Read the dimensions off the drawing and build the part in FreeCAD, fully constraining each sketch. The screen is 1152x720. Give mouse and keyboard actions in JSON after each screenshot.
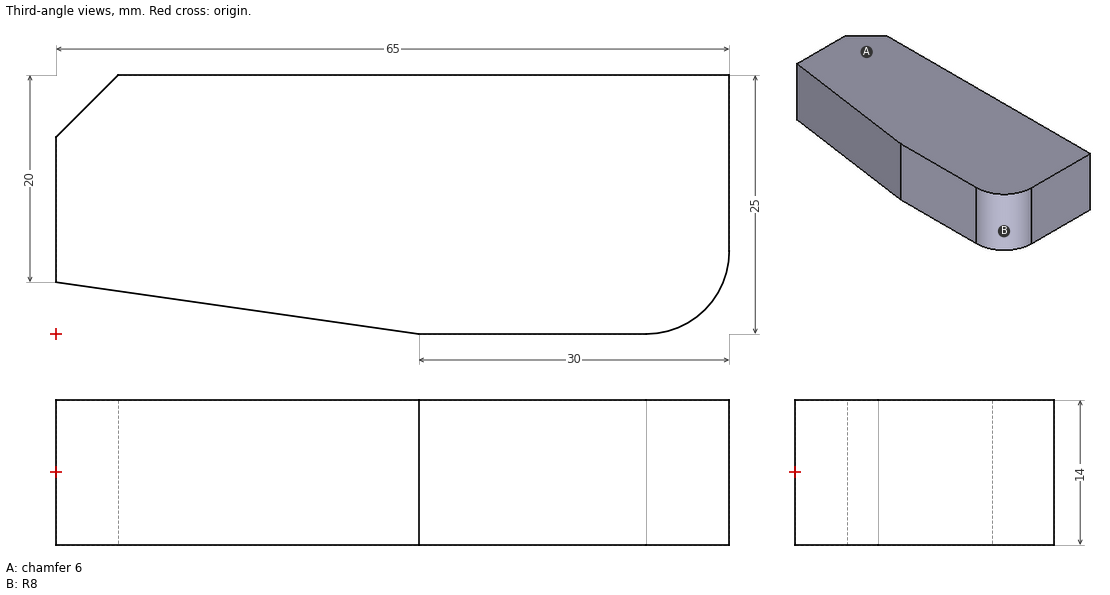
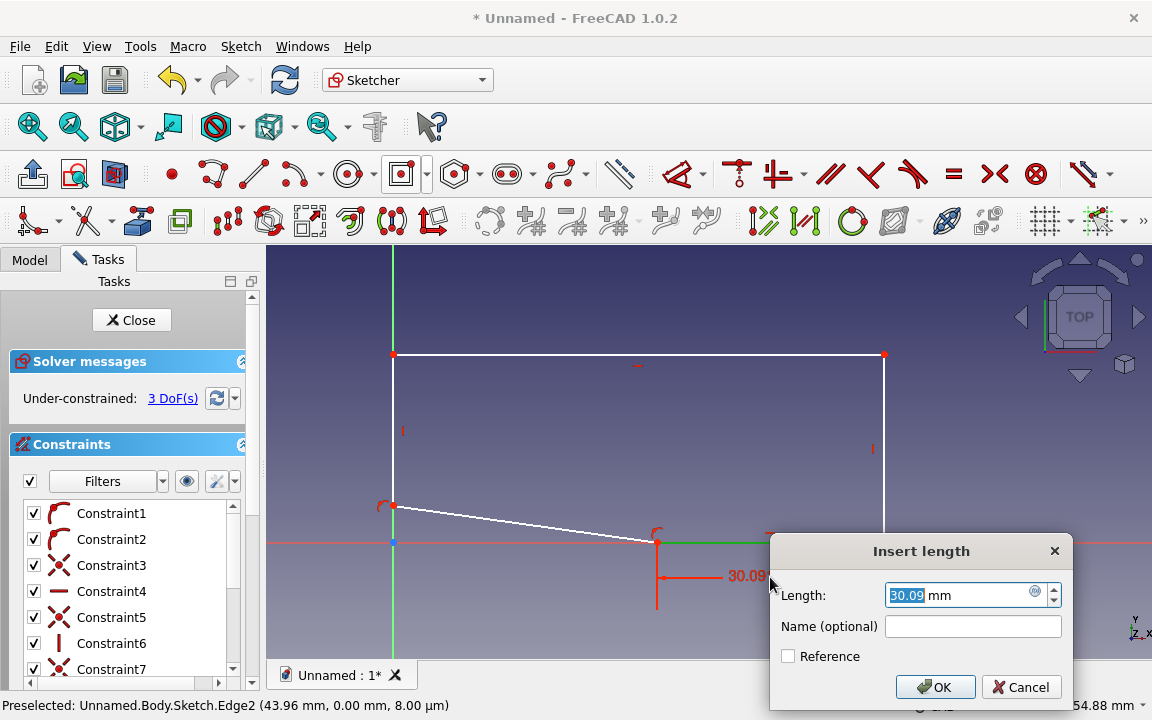
{"action": "type", "text": "30"}
{"action": "key", "text": "Return"}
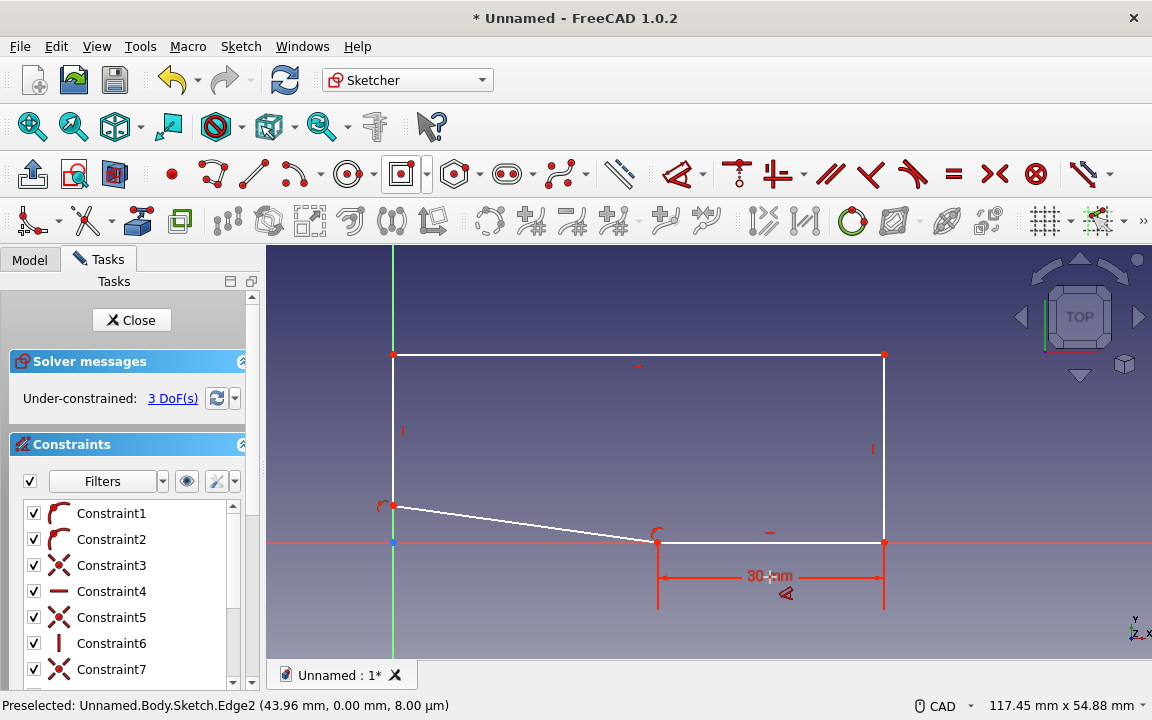
{"action": "left_click", "coordinate": [884, 486]}
{"action": "left_click", "coordinate": [918, 449]}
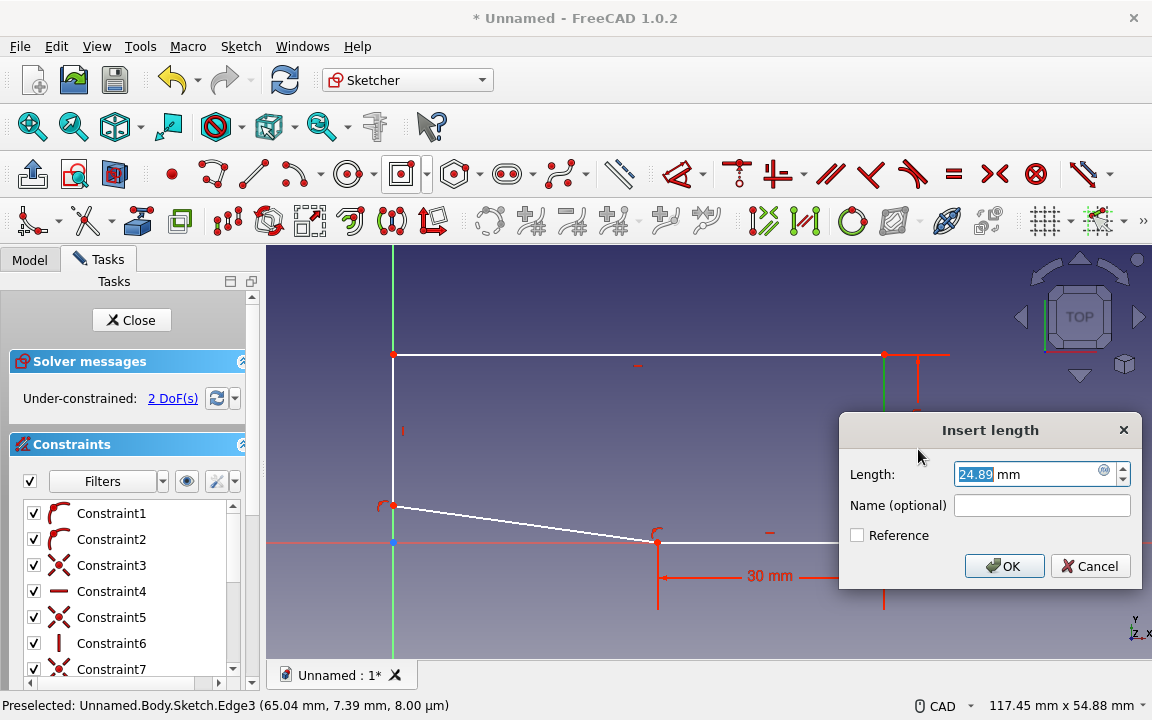
{"action": "type", "text": "25"}
{"action": "key", "text": "Return"}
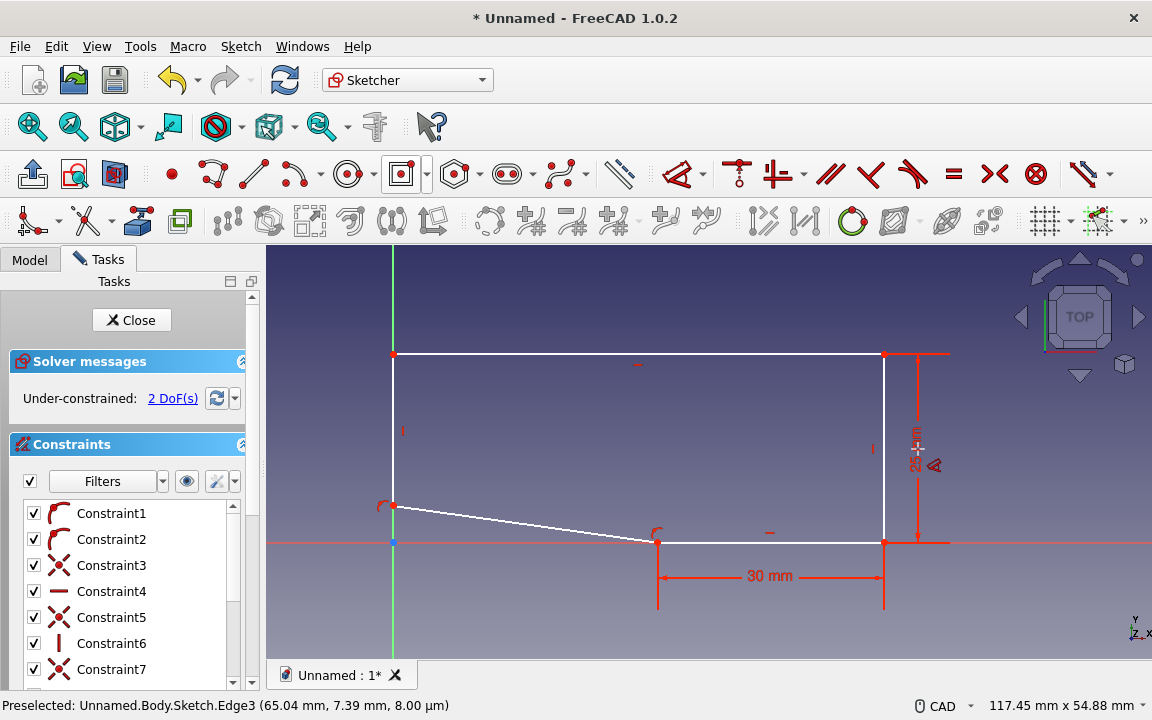
{"action": "left_click", "coordinate": [737, 354]}
{"action": "left_click", "coordinate": [639, 320]}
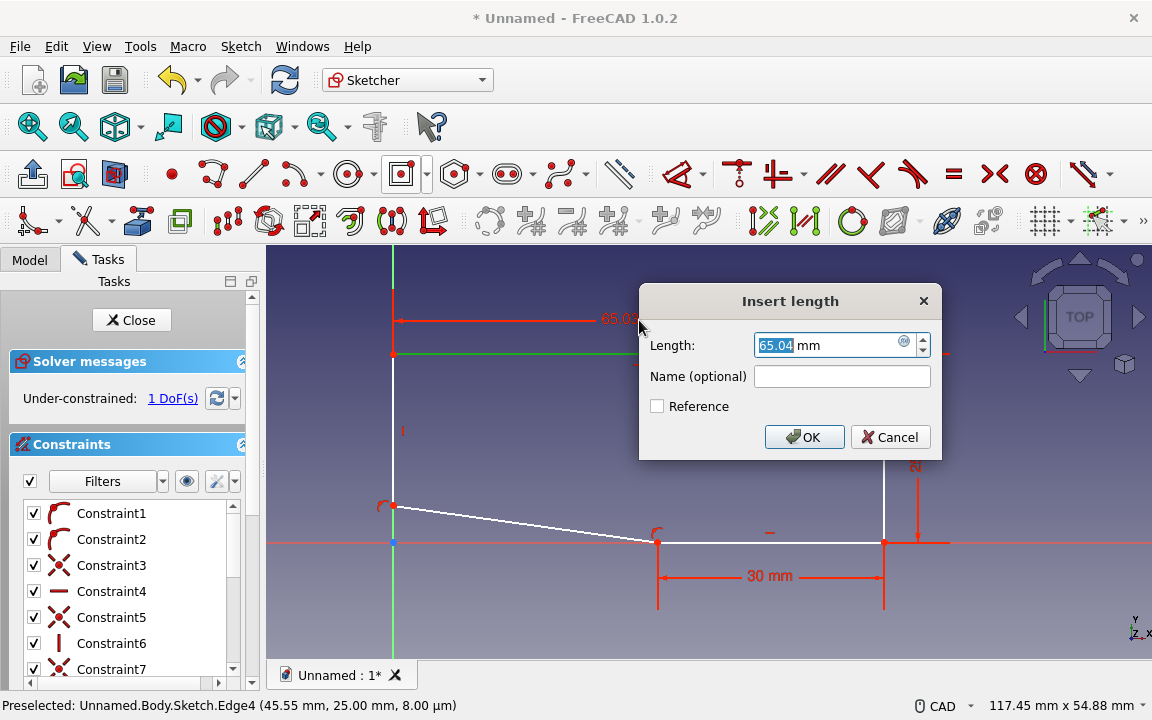
{"action": "type", "text": "65"}
{"action": "key", "text": "Return"}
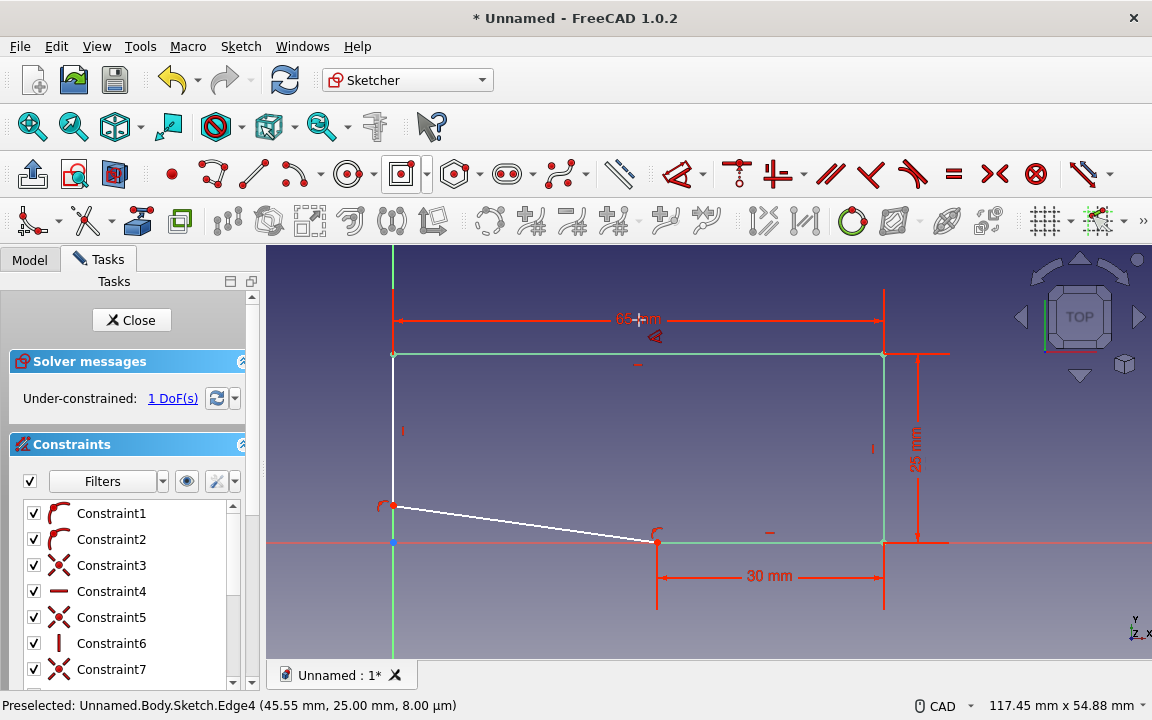
{"action": "left_click", "coordinate": [393, 400]}
{"action": "left_click", "coordinate": [359, 430]}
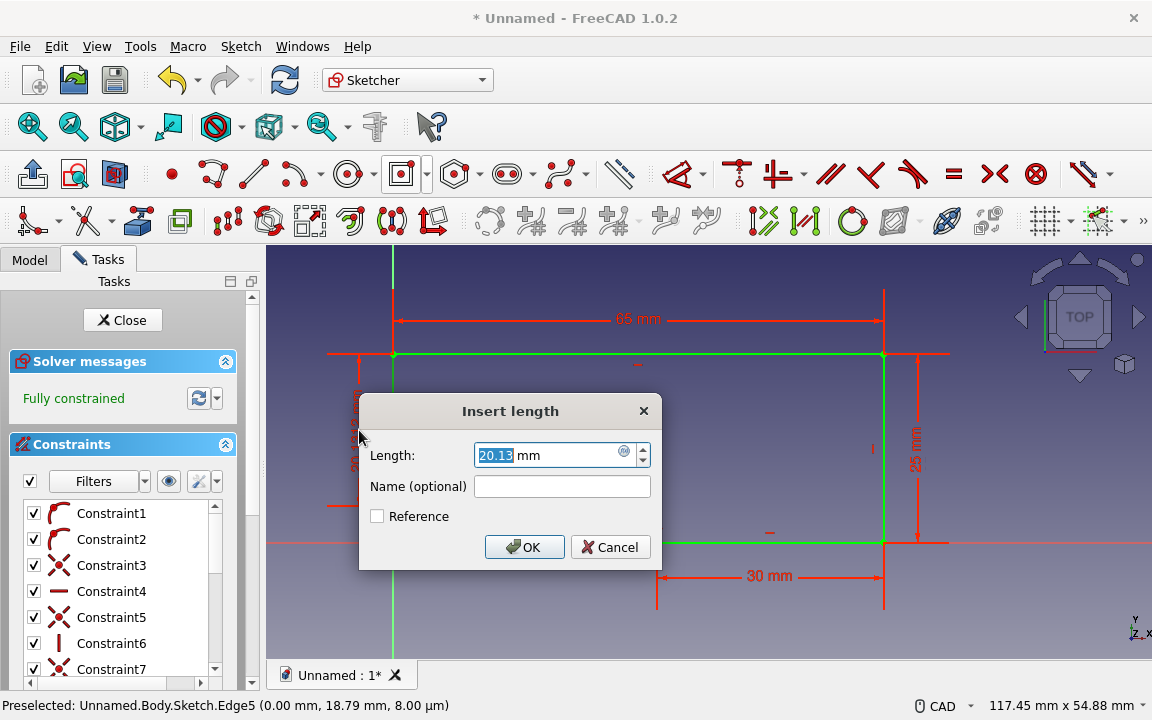
{"action": "type", "text": "20"}
{"action": "key", "text": "Return"}
{"action": "key", "text": "Escape"}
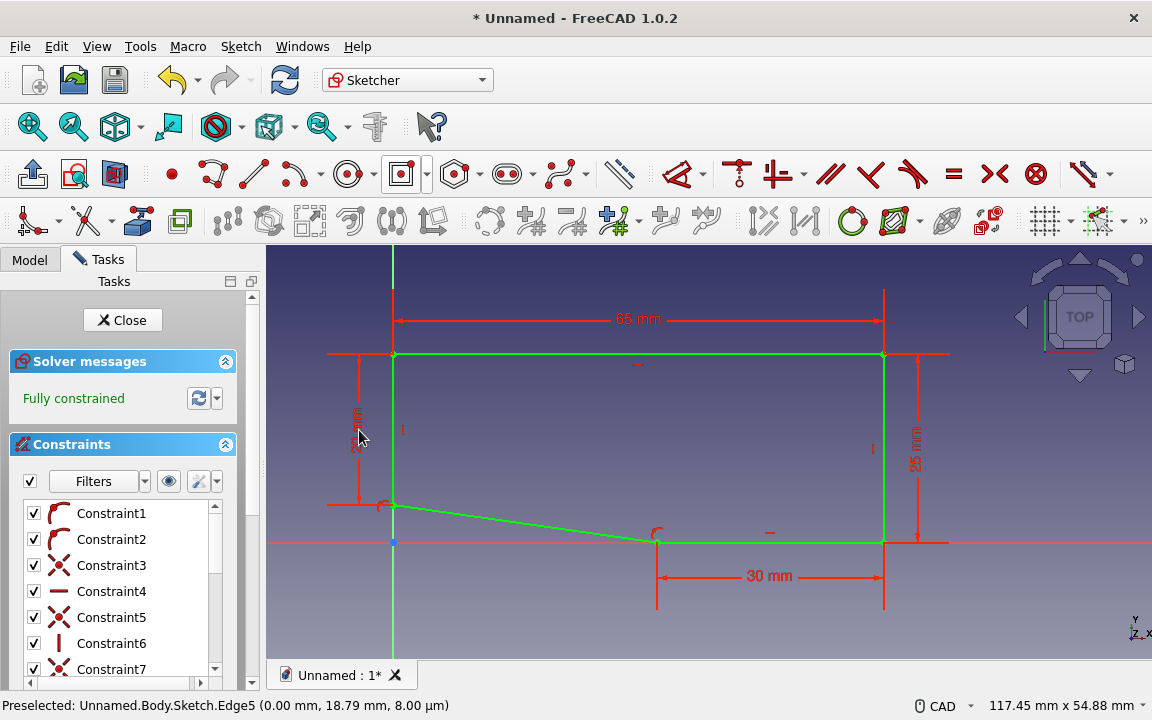
{"action": "left_click", "coordinate": [123, 320]}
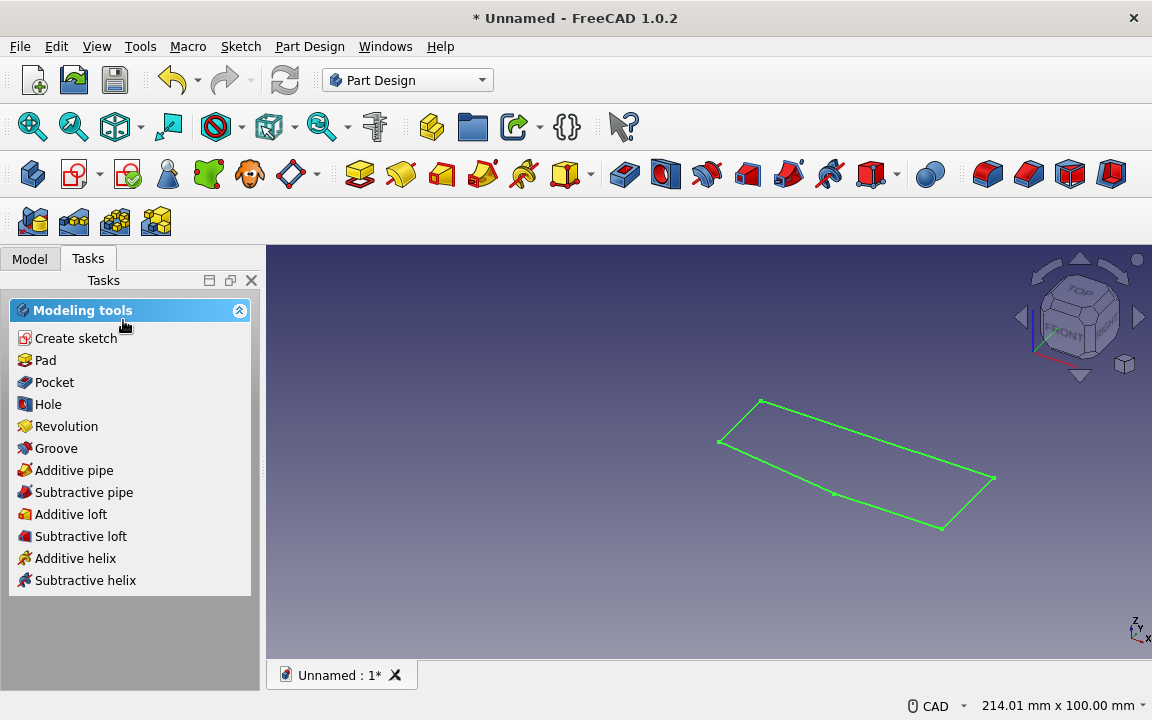
{"action": "left_click", "coordinate": [360, 174]}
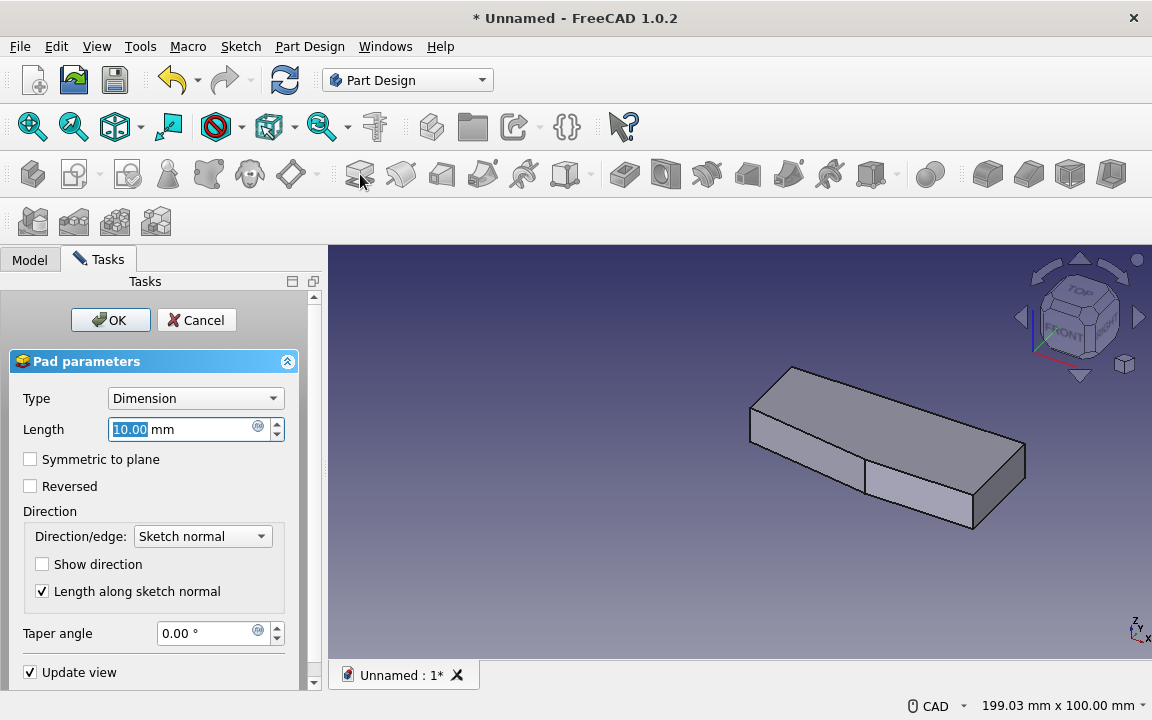
{"action": "type", "text": "14"}
{"action": "key", "text": "Tab"}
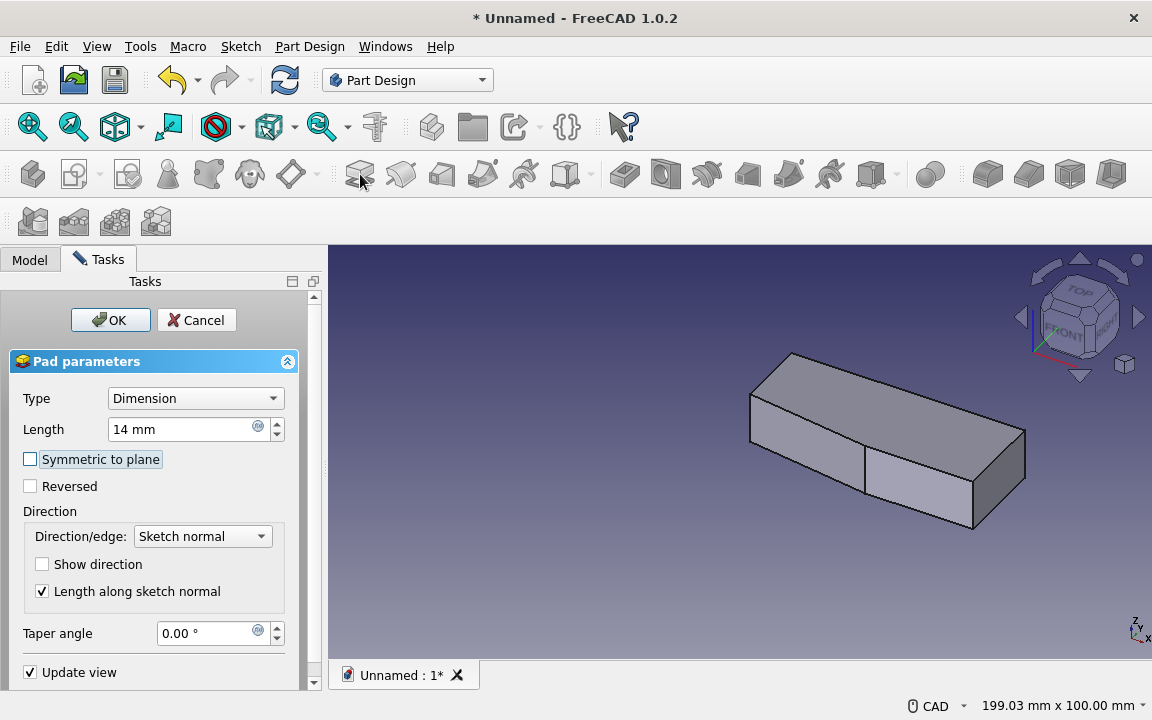
{"action": "left_click", "coordinate": [31, 459]}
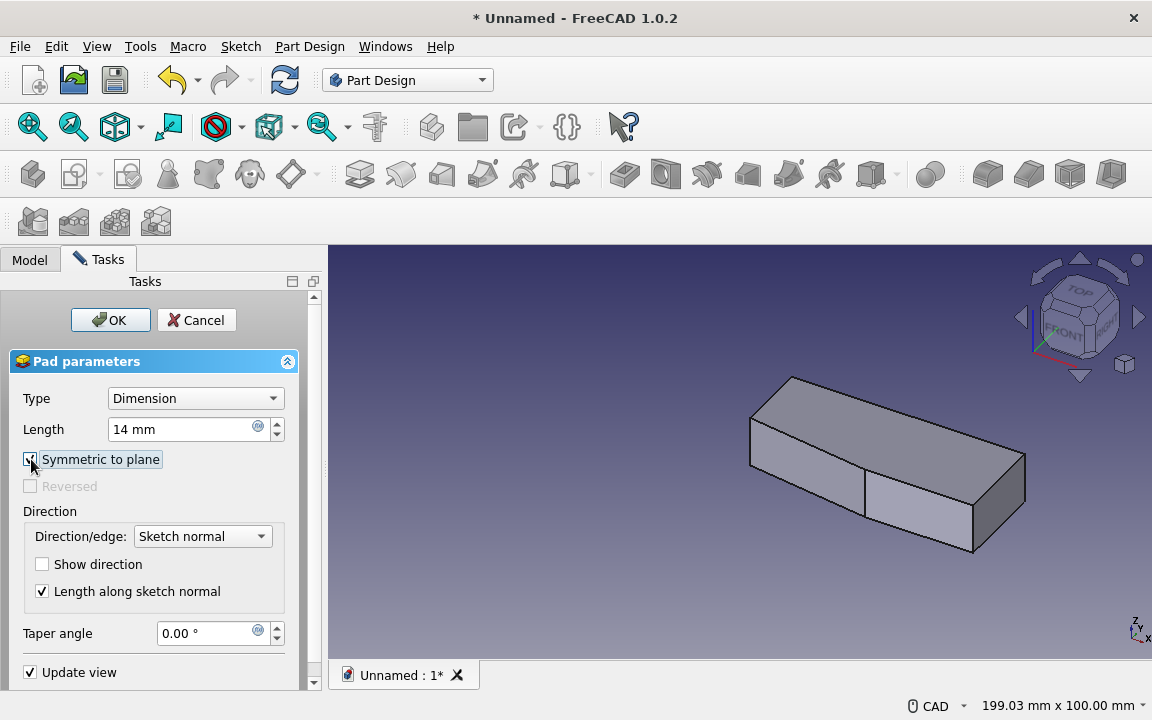
{"action": "left_click", "coordinate": [111, 320]}